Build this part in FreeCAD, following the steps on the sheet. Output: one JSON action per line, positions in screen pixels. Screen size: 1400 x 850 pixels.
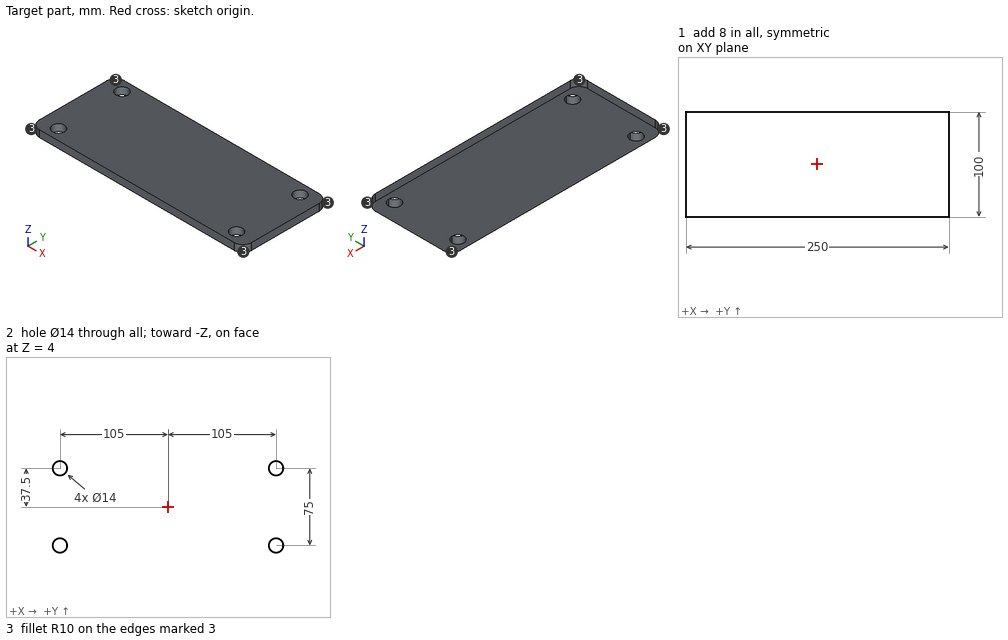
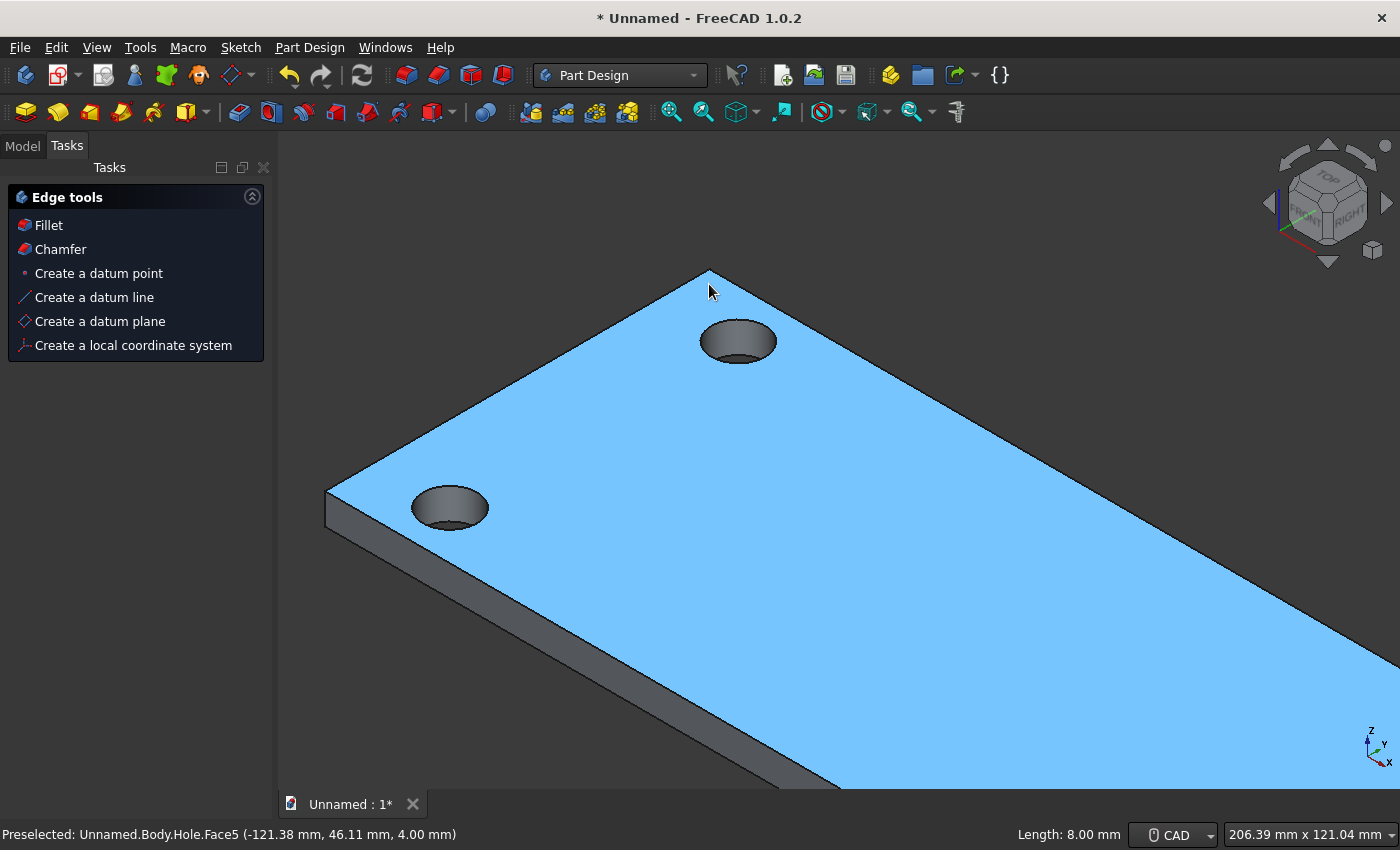
{"action": "left_click", "coordinate": [672, 112]}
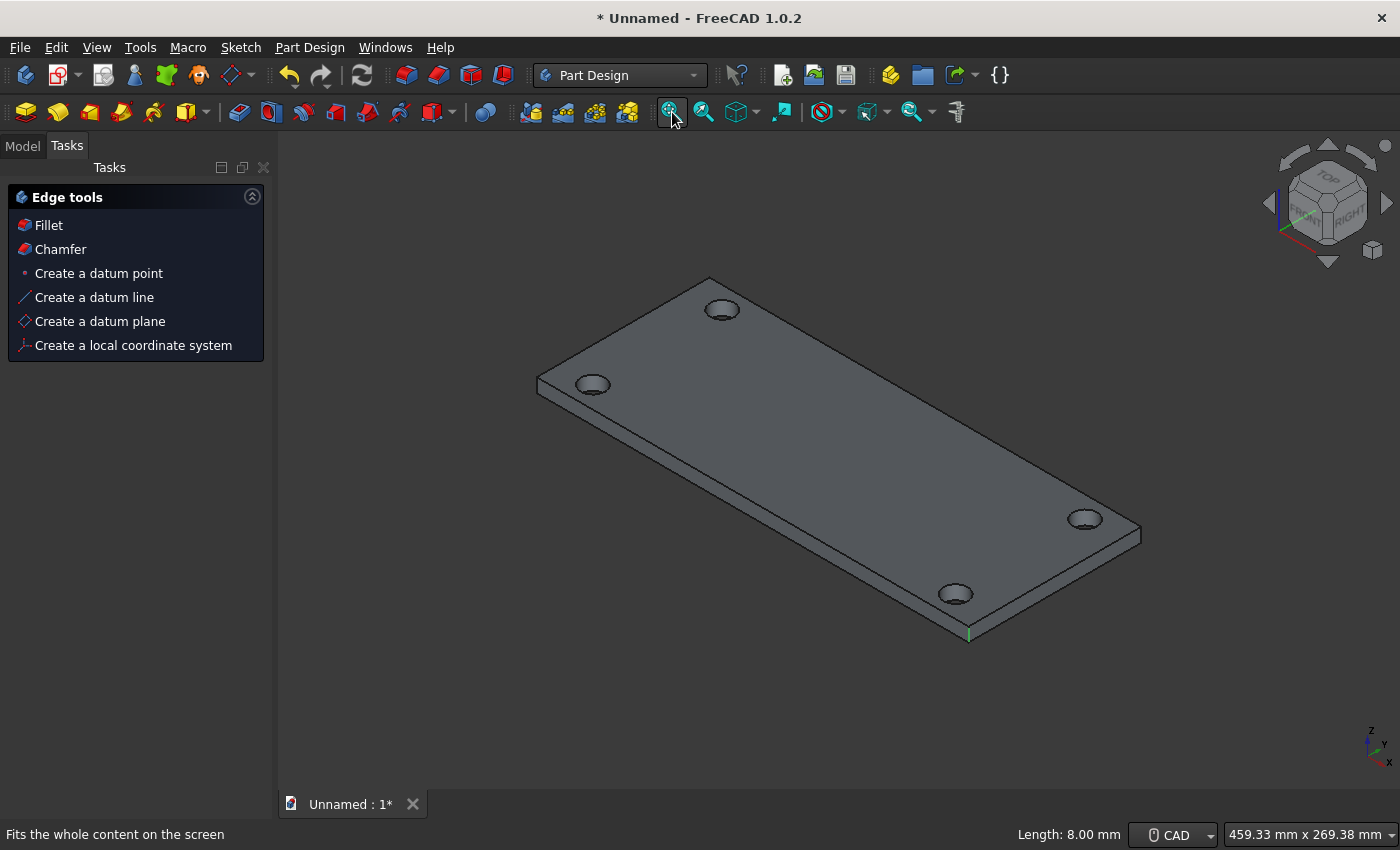
{"action": "key", "text": "2"}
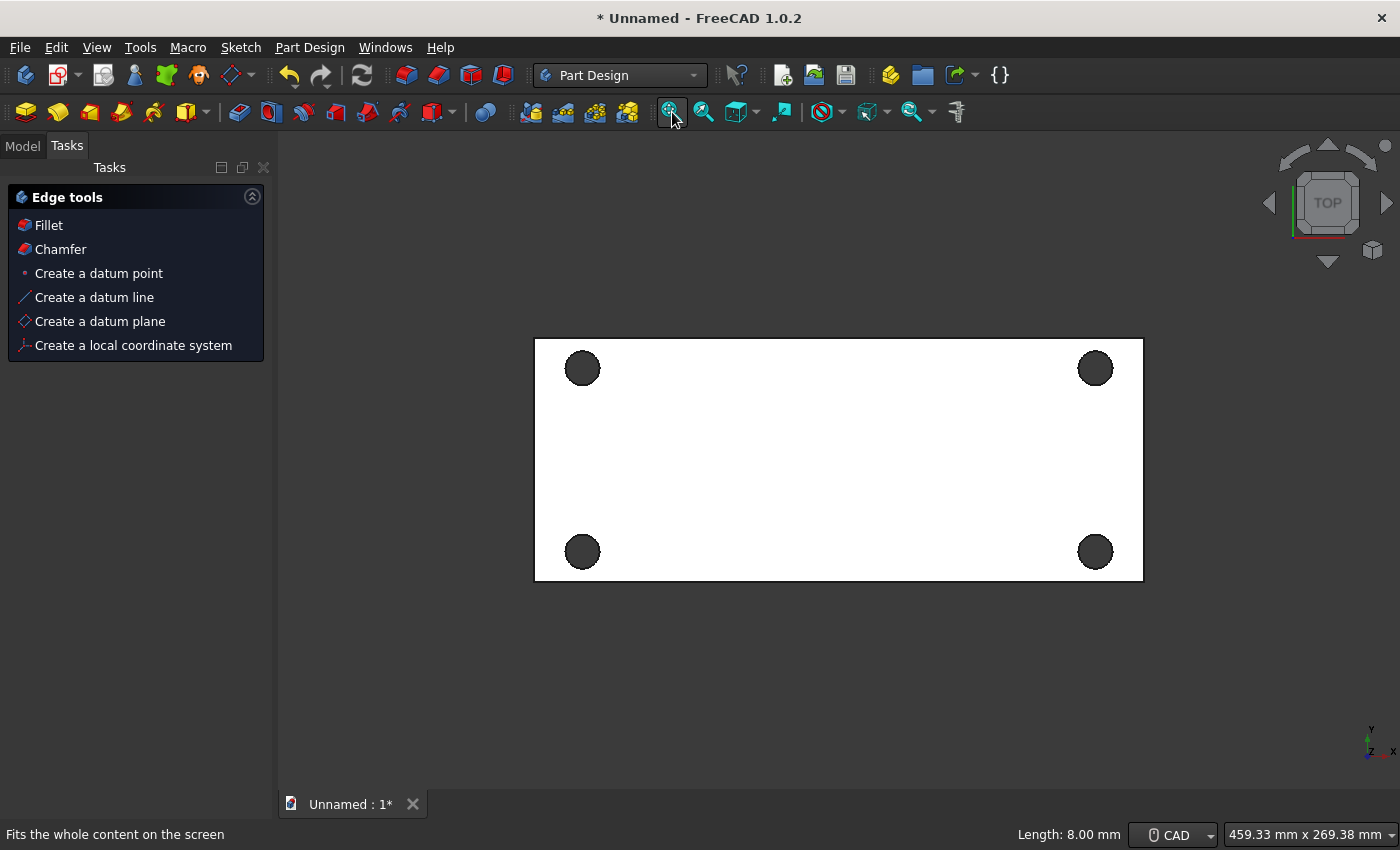
{"action": "scroll", "coordinate": [534, 337], "scroll_direction": "up", "scroll_amount": 4}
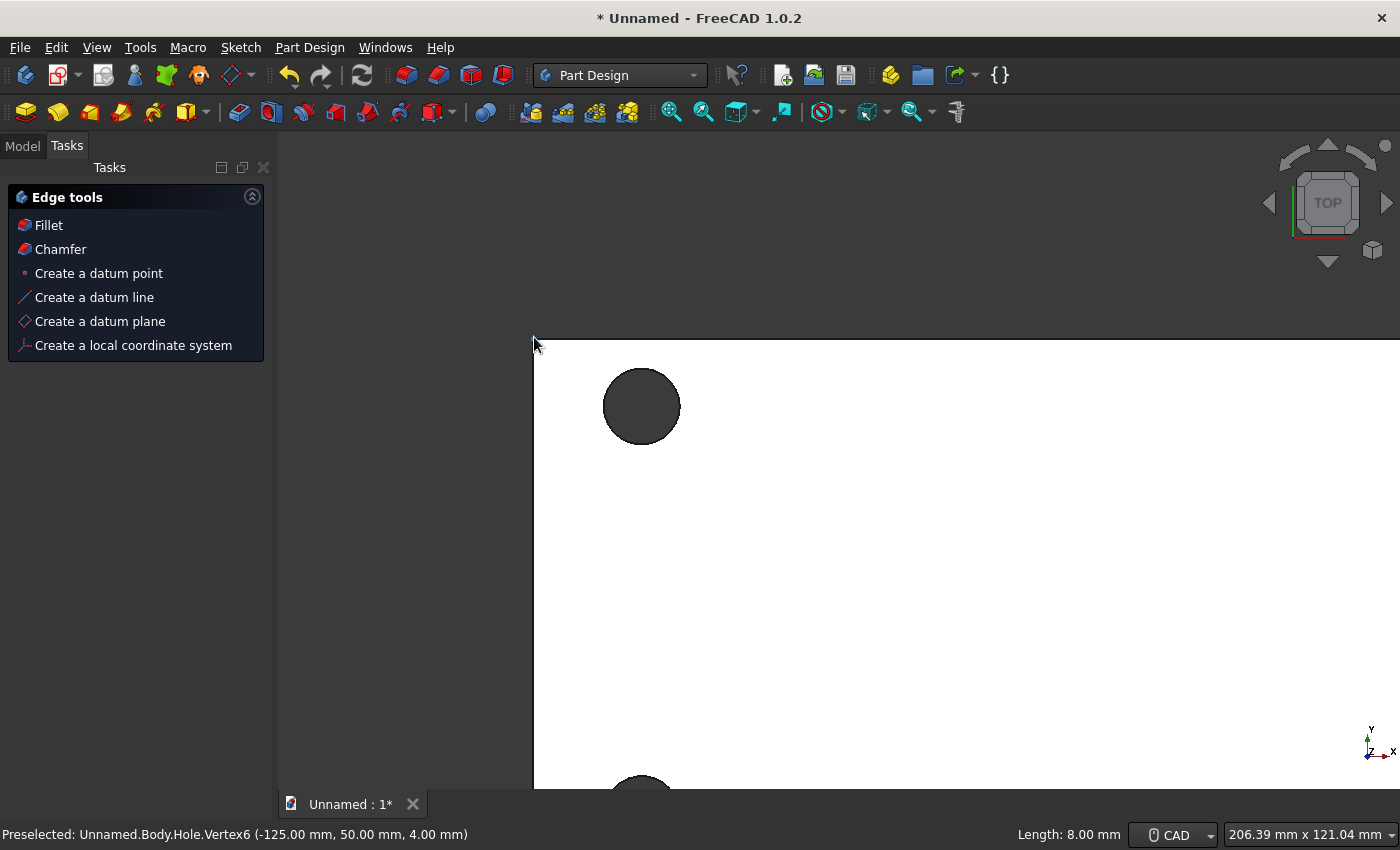
{"action": "left_click", "coordinate": [672, 112]}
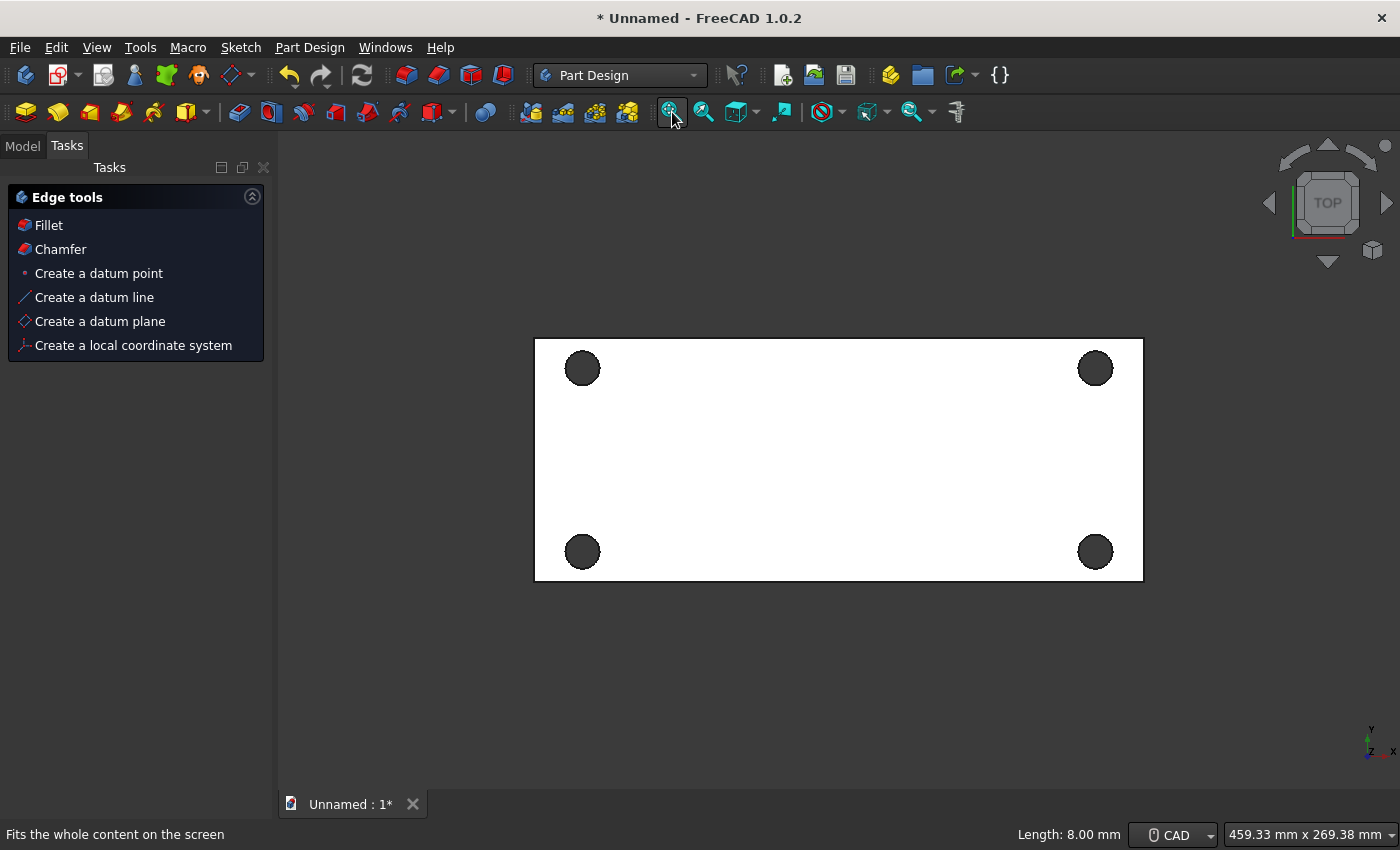
{"action": "key", "text": "1"}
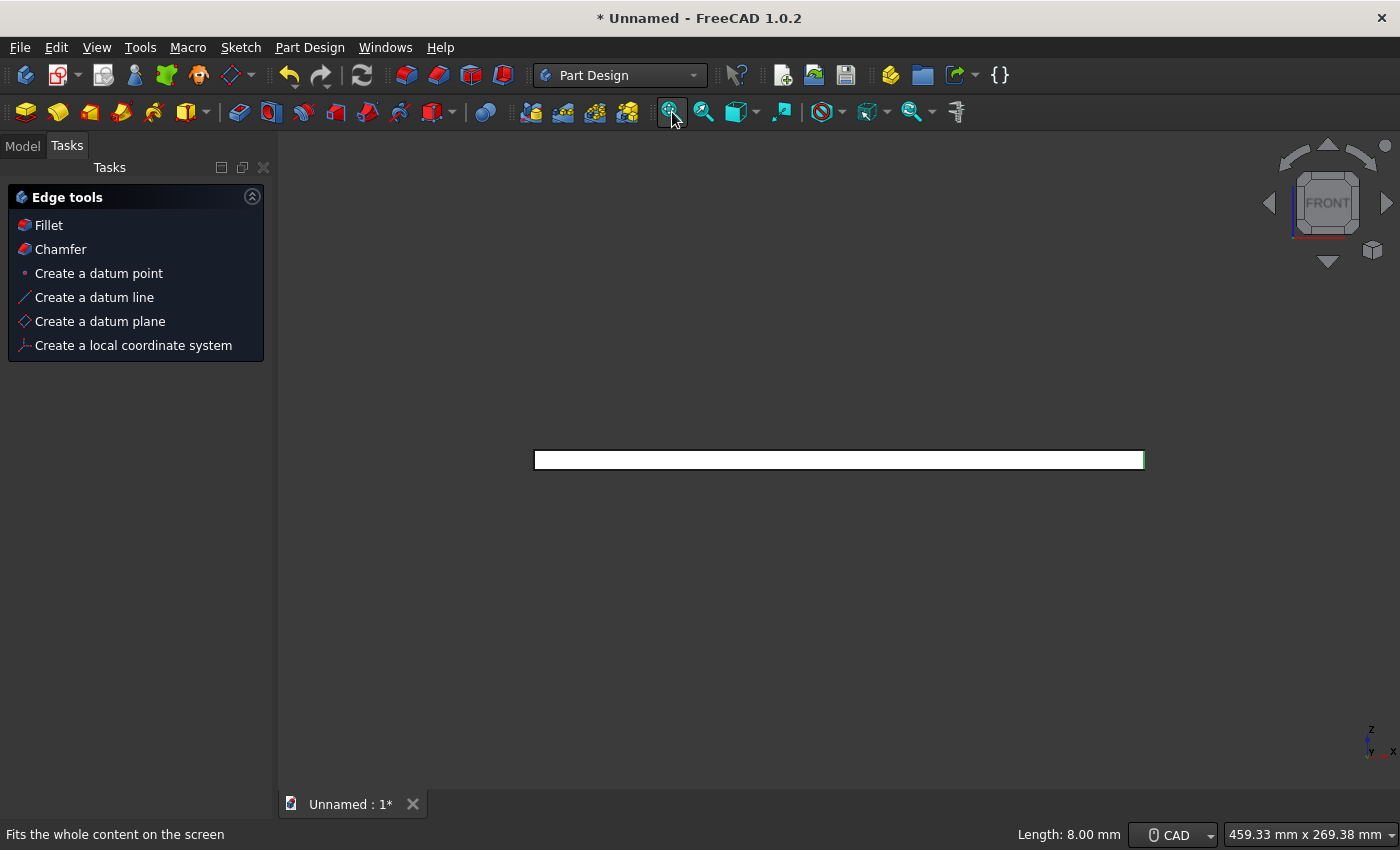
{"action": "left_click", "coordinate": [534, 459], "text": "ctrl"}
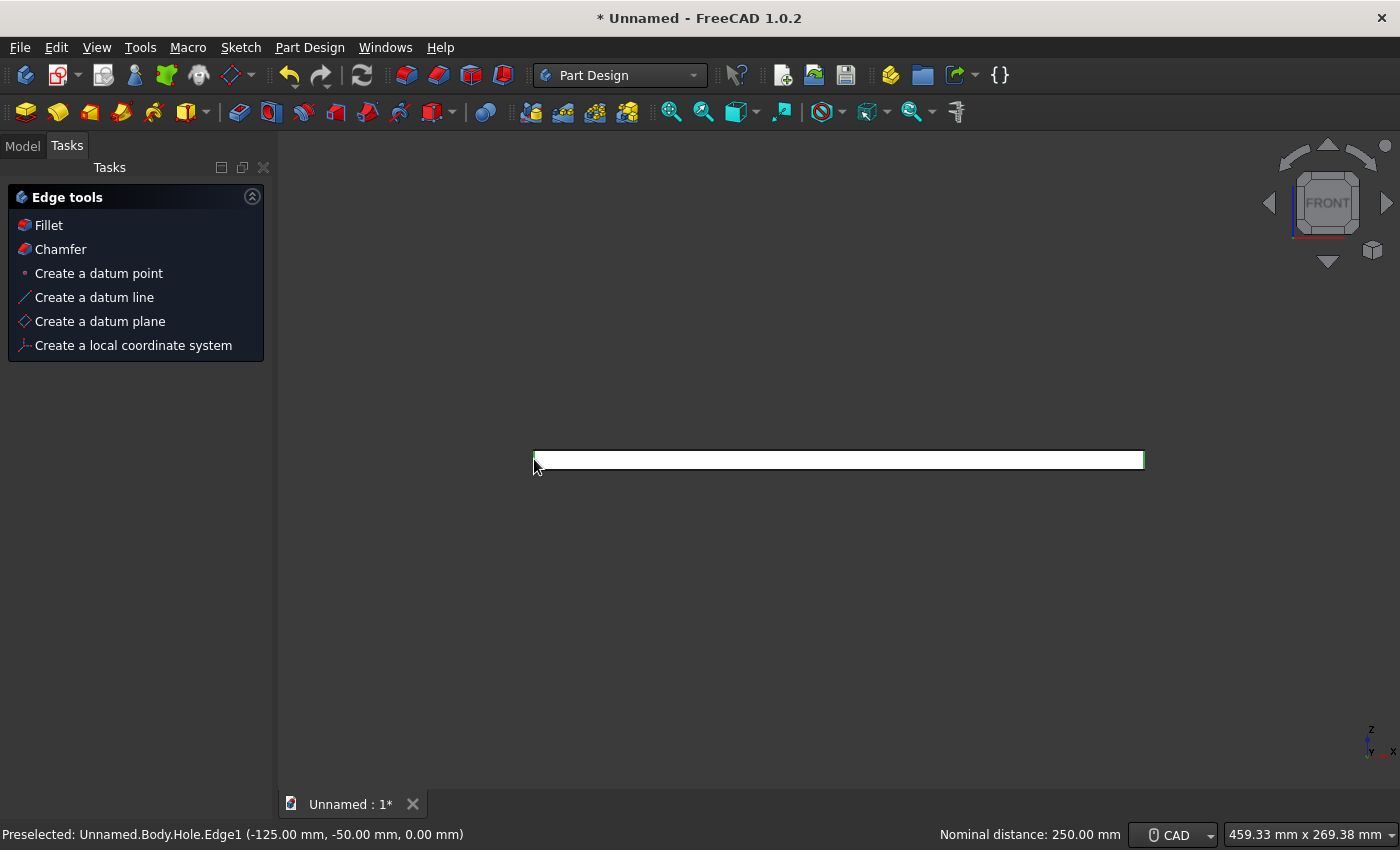
{"action": "scroll", "coordinate": [534, 459], "scroll_direction": "up", "scroll_amount": 4}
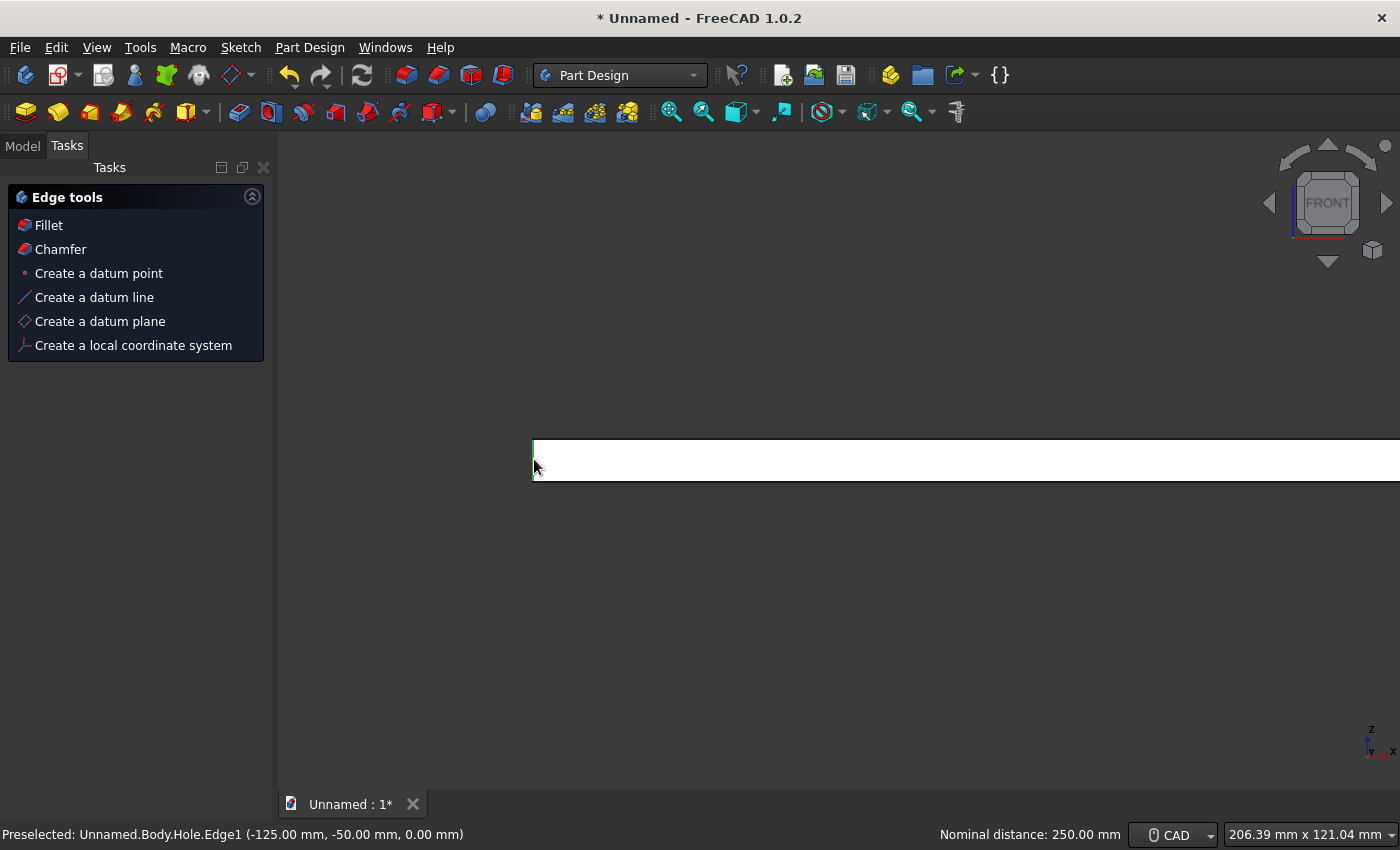
{"action": "left_click", "coordinate": [672, 112]}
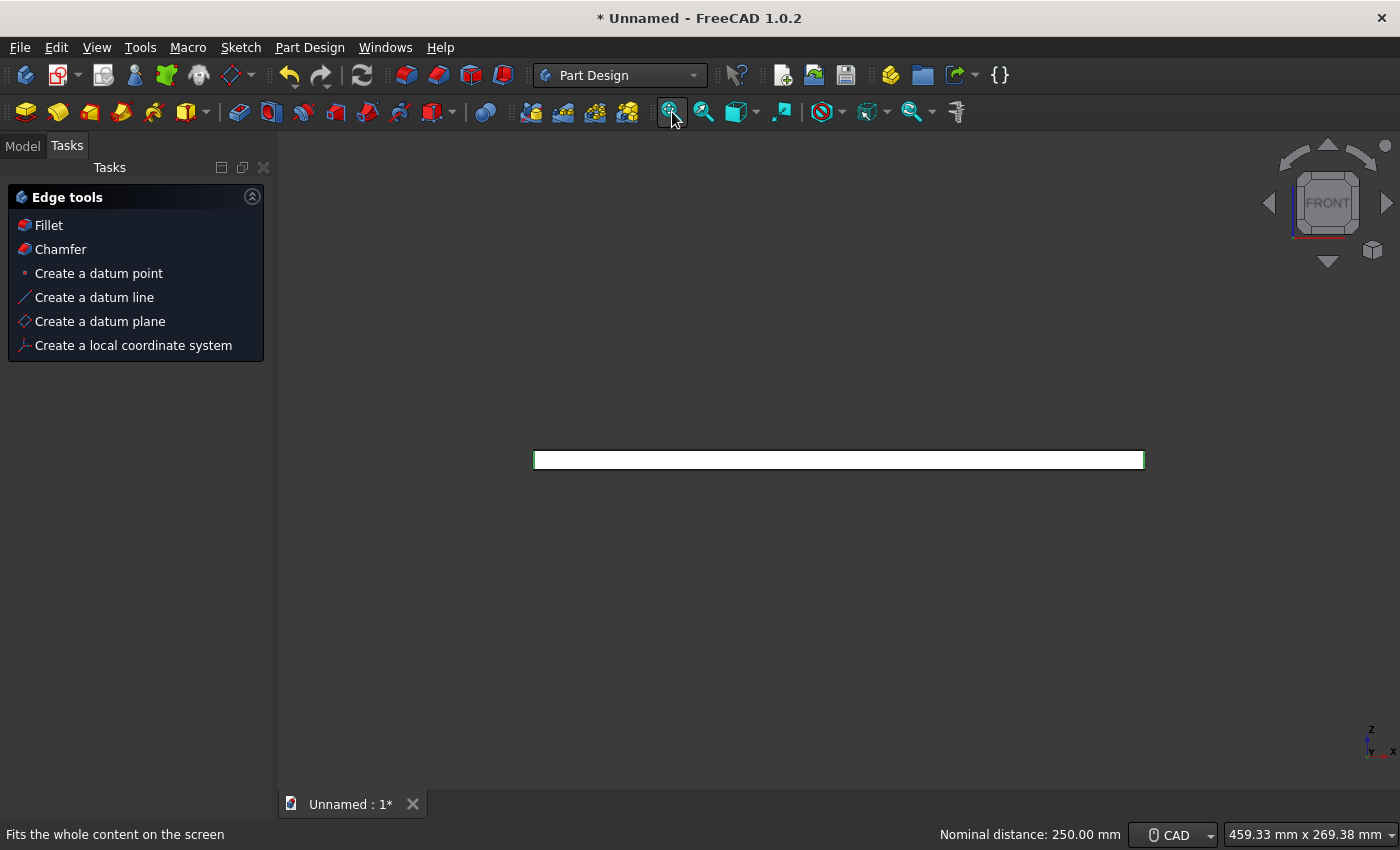
{"action": "key", "text": "3"}